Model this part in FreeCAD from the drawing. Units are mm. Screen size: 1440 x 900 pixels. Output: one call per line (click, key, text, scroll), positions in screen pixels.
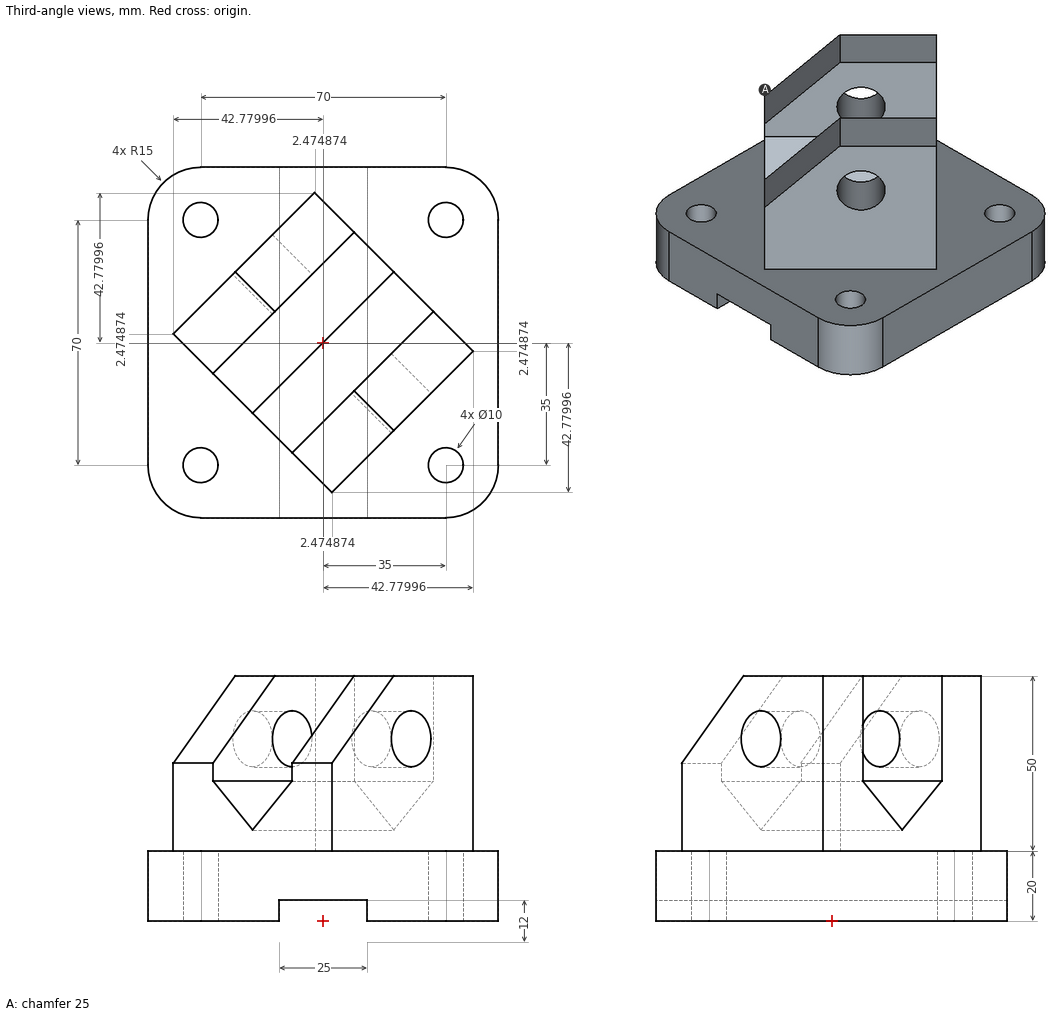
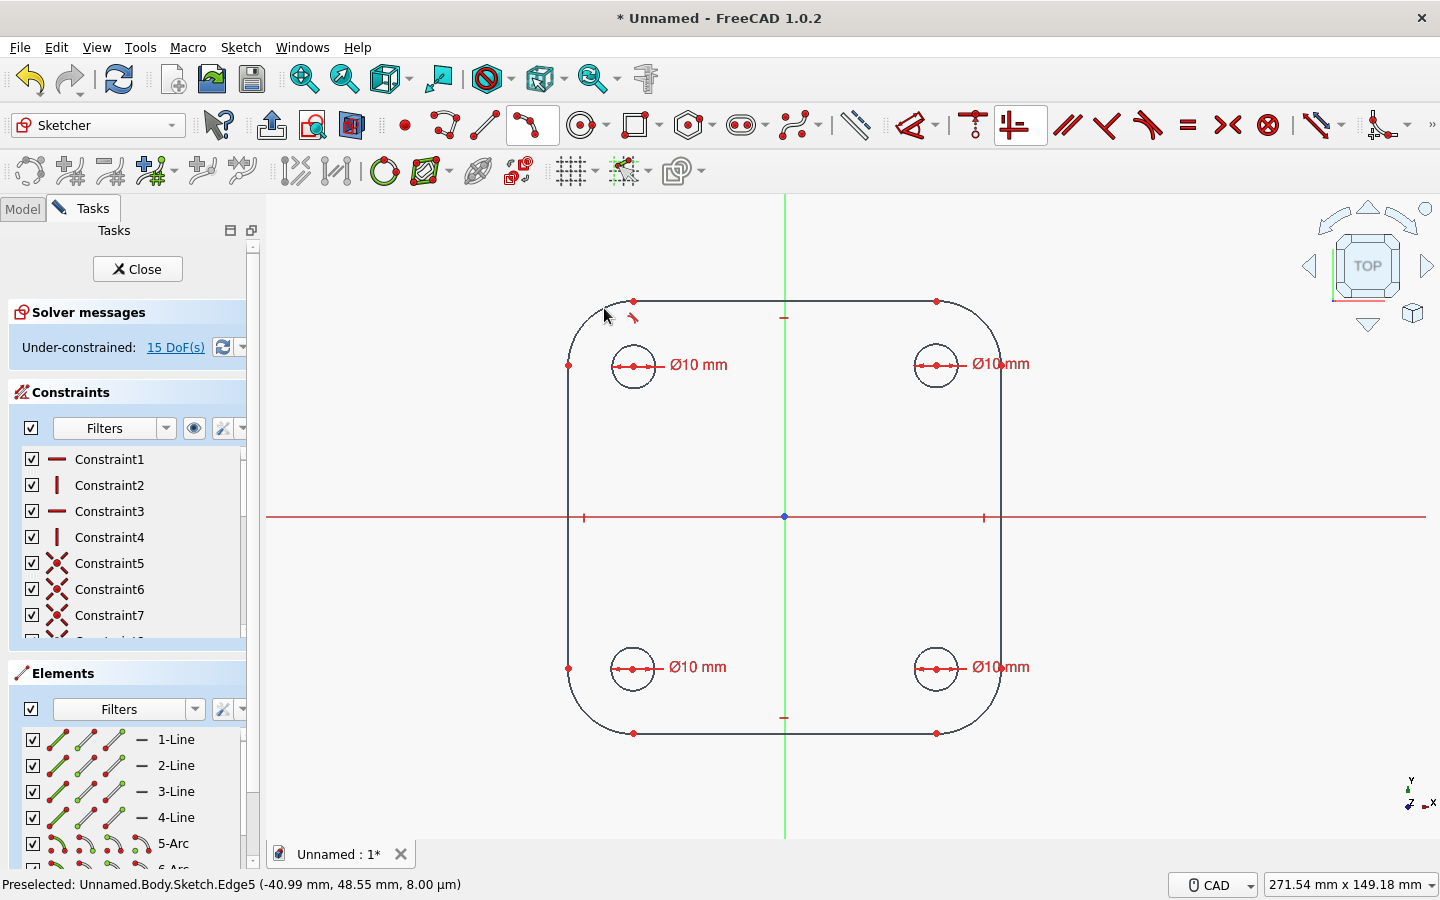
click(845, 301)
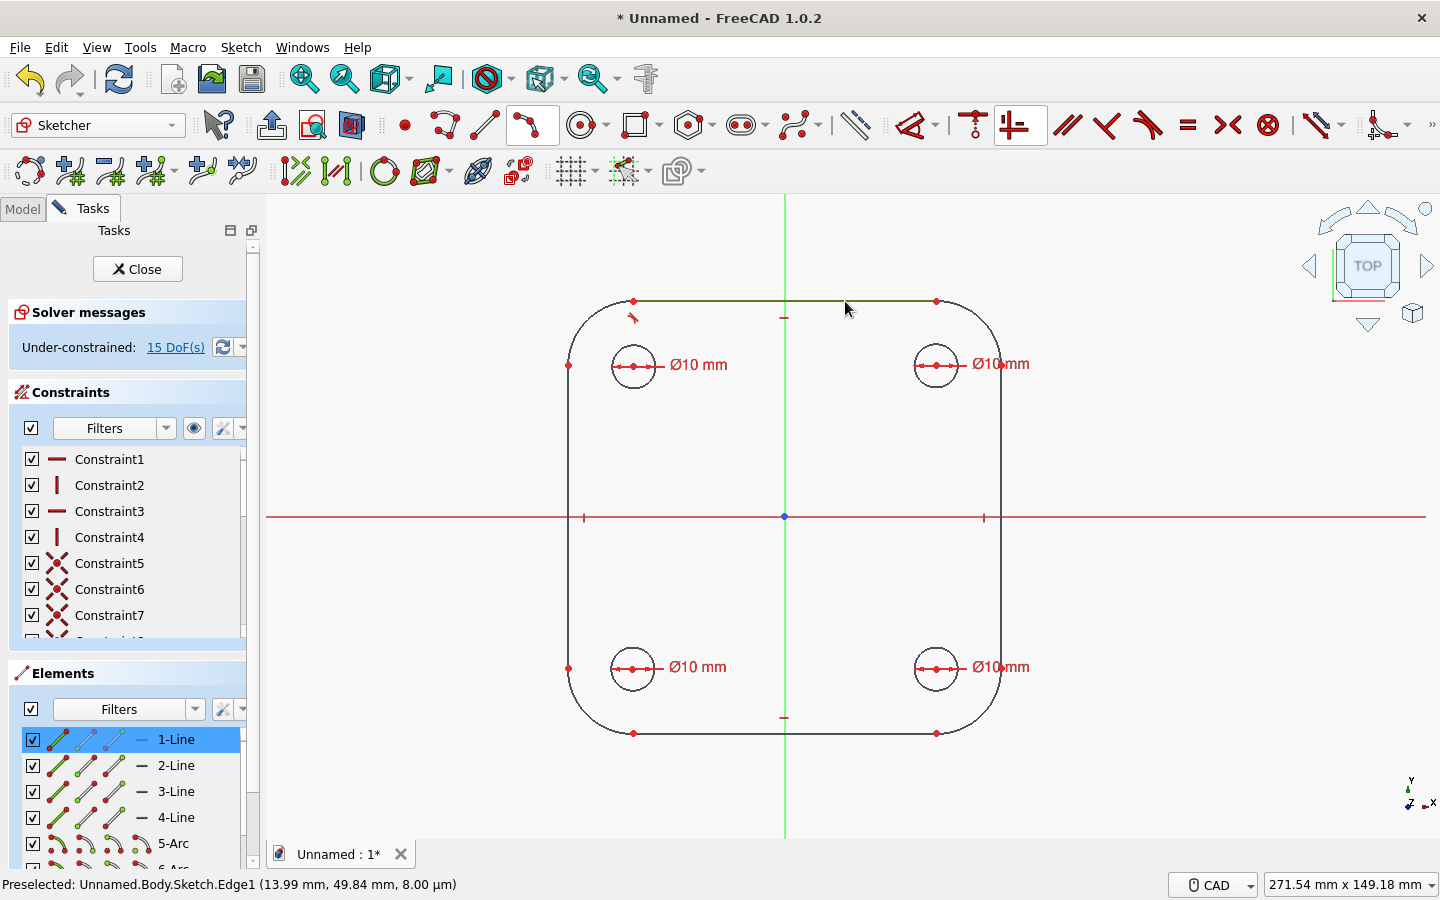
click(994, 336)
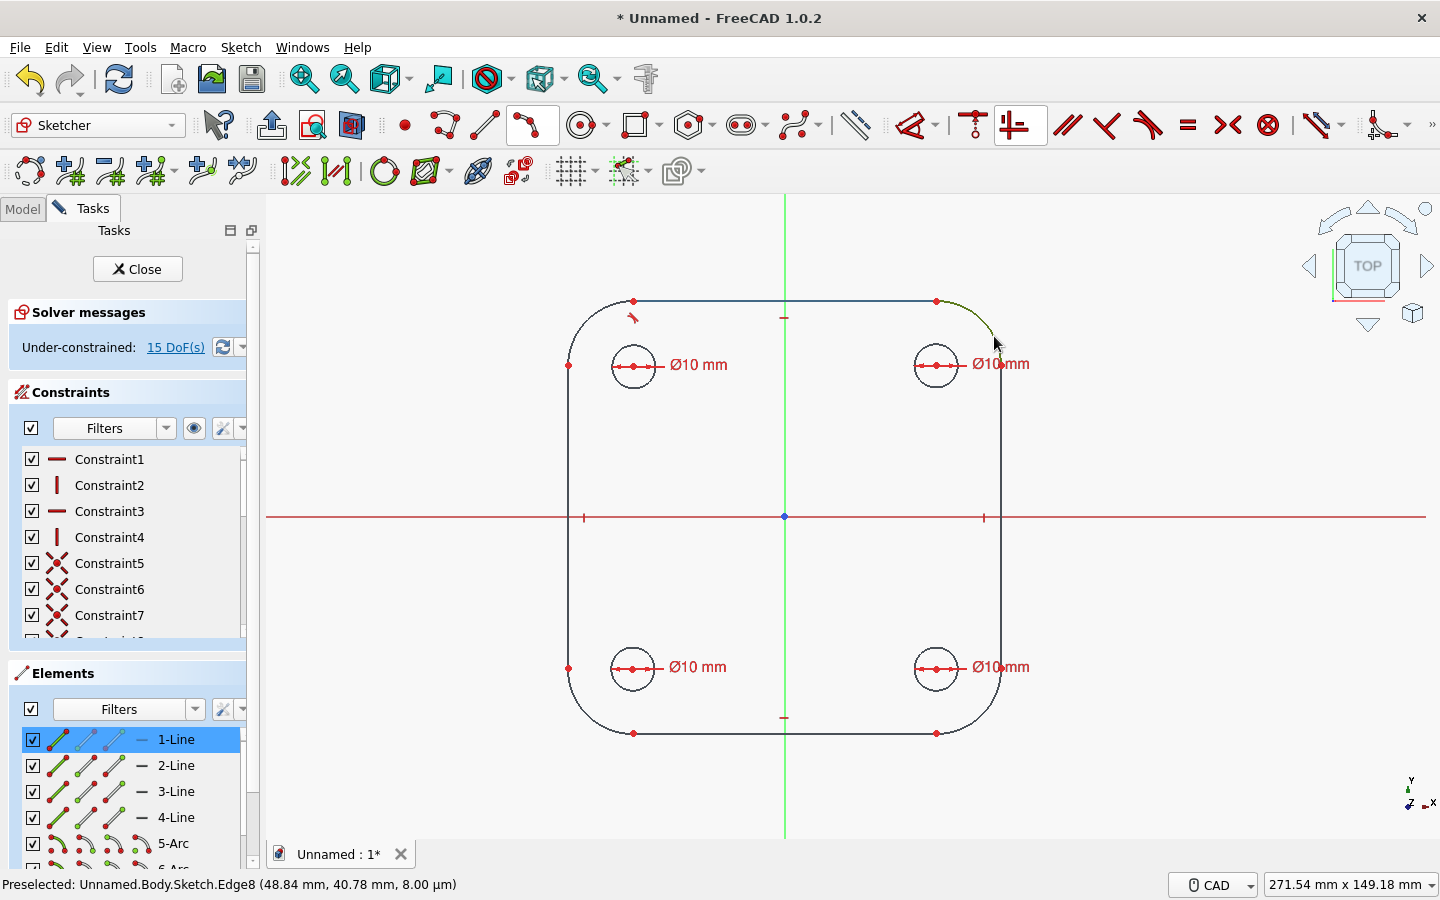
click(1148, 126)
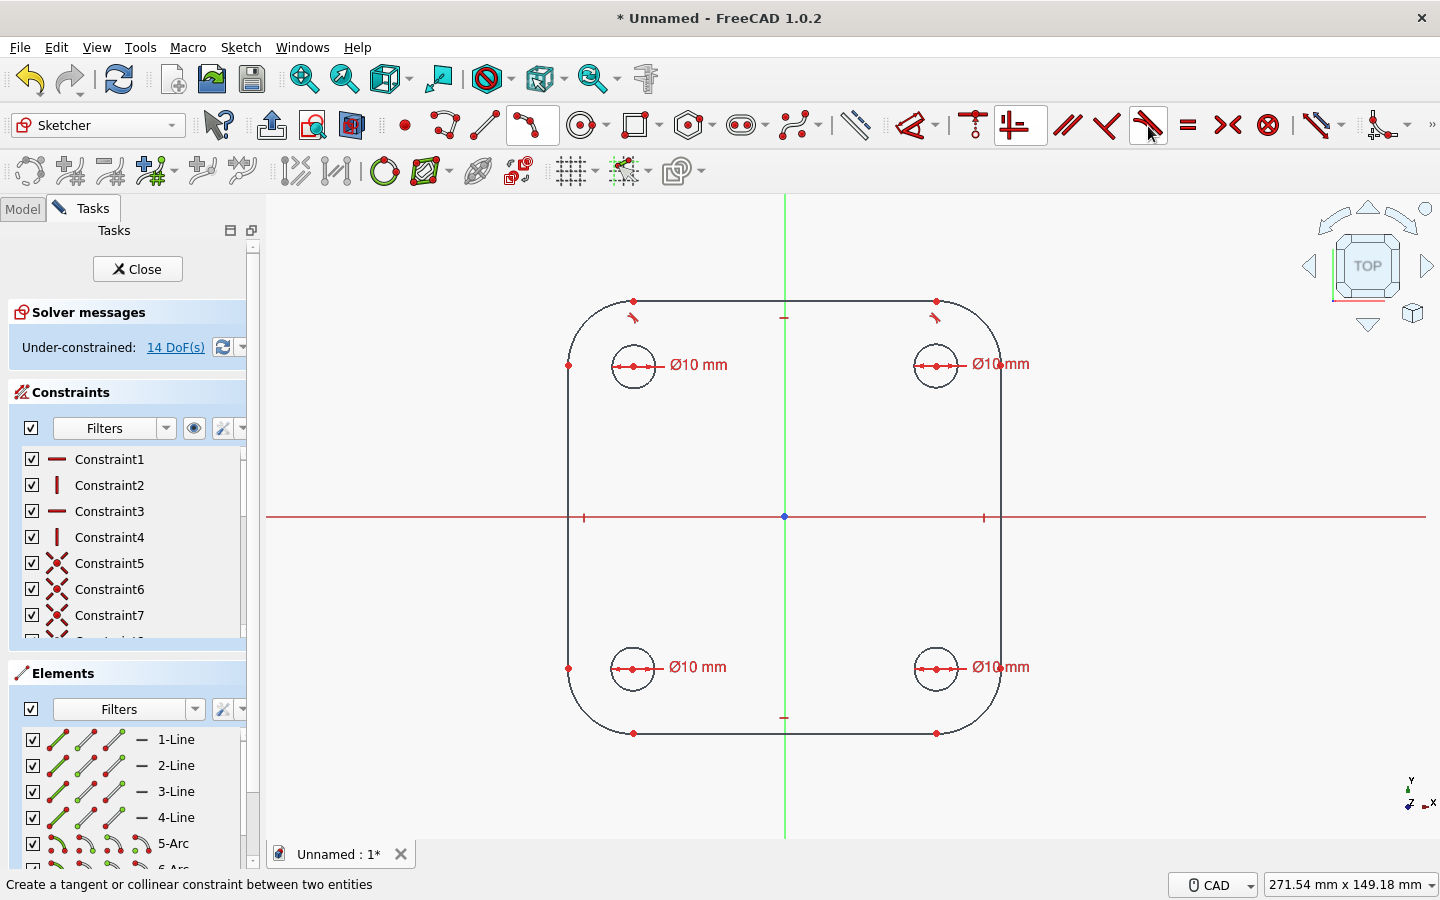
click(568, 457)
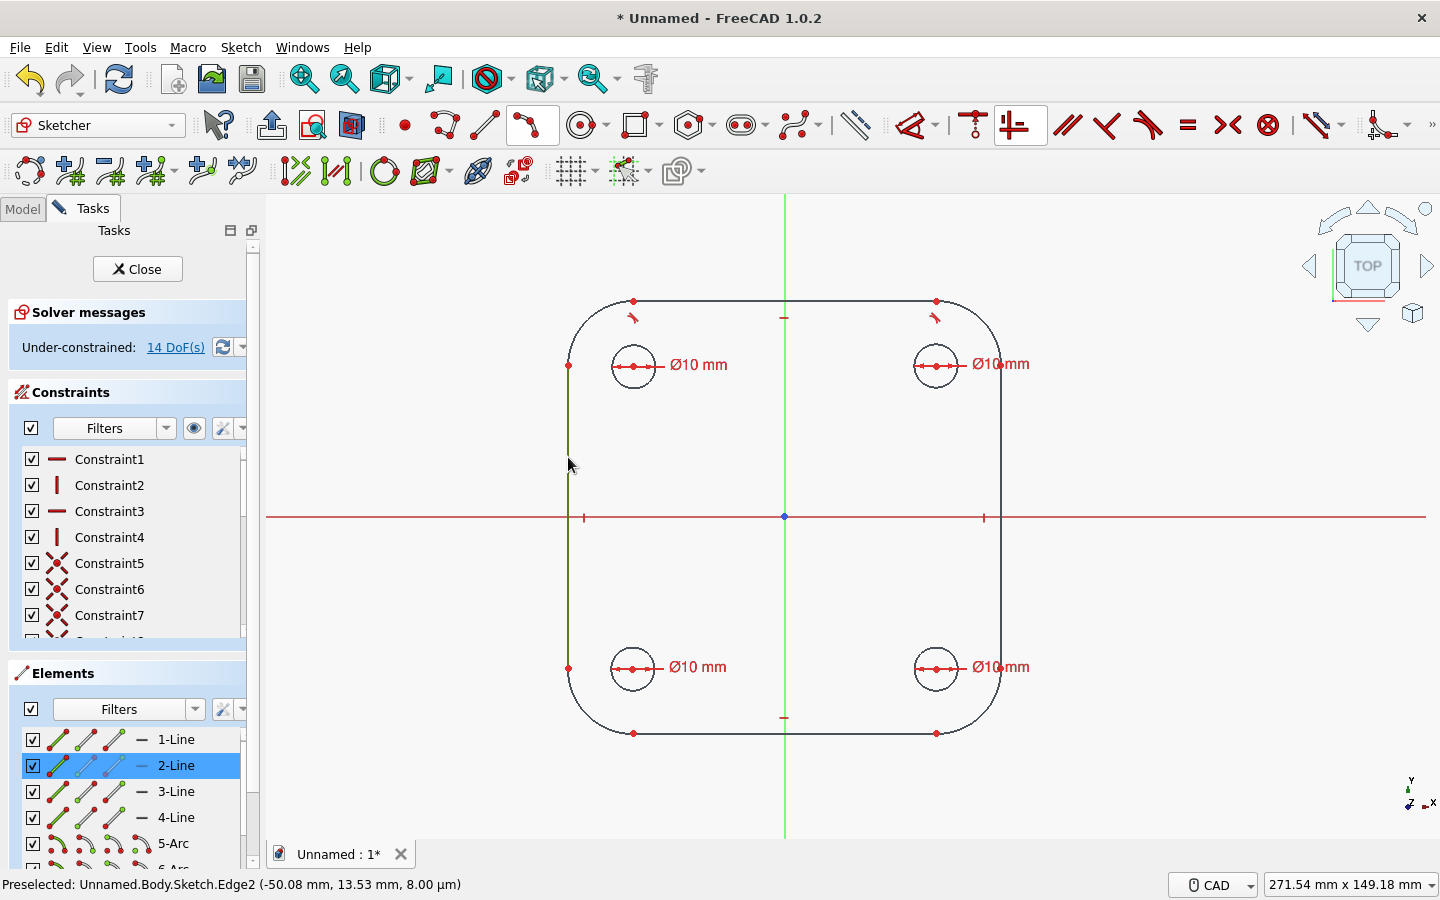
click(604, 308)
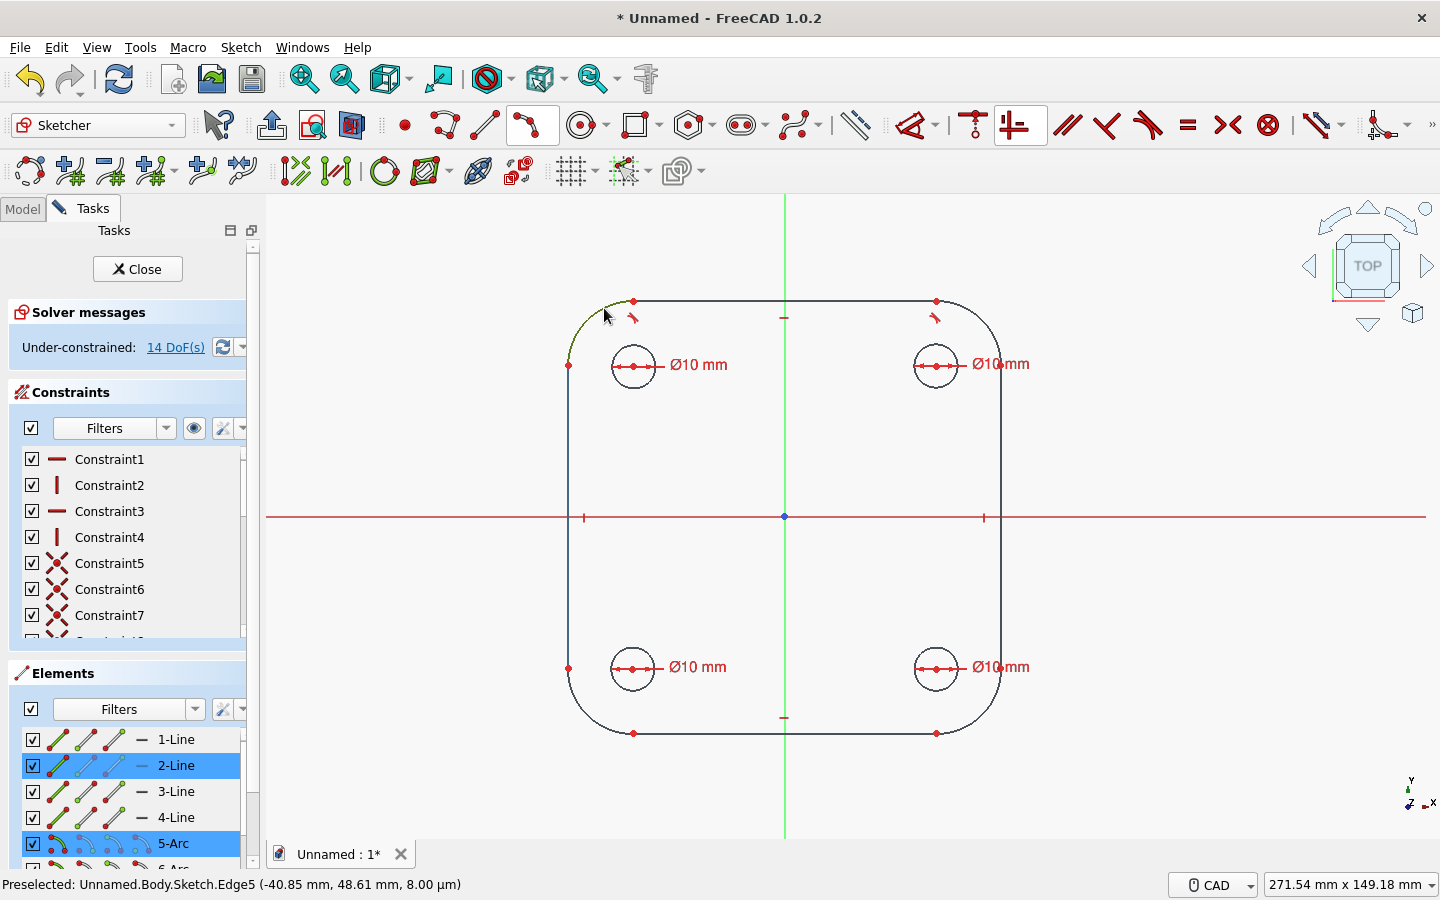
click(1148, 126)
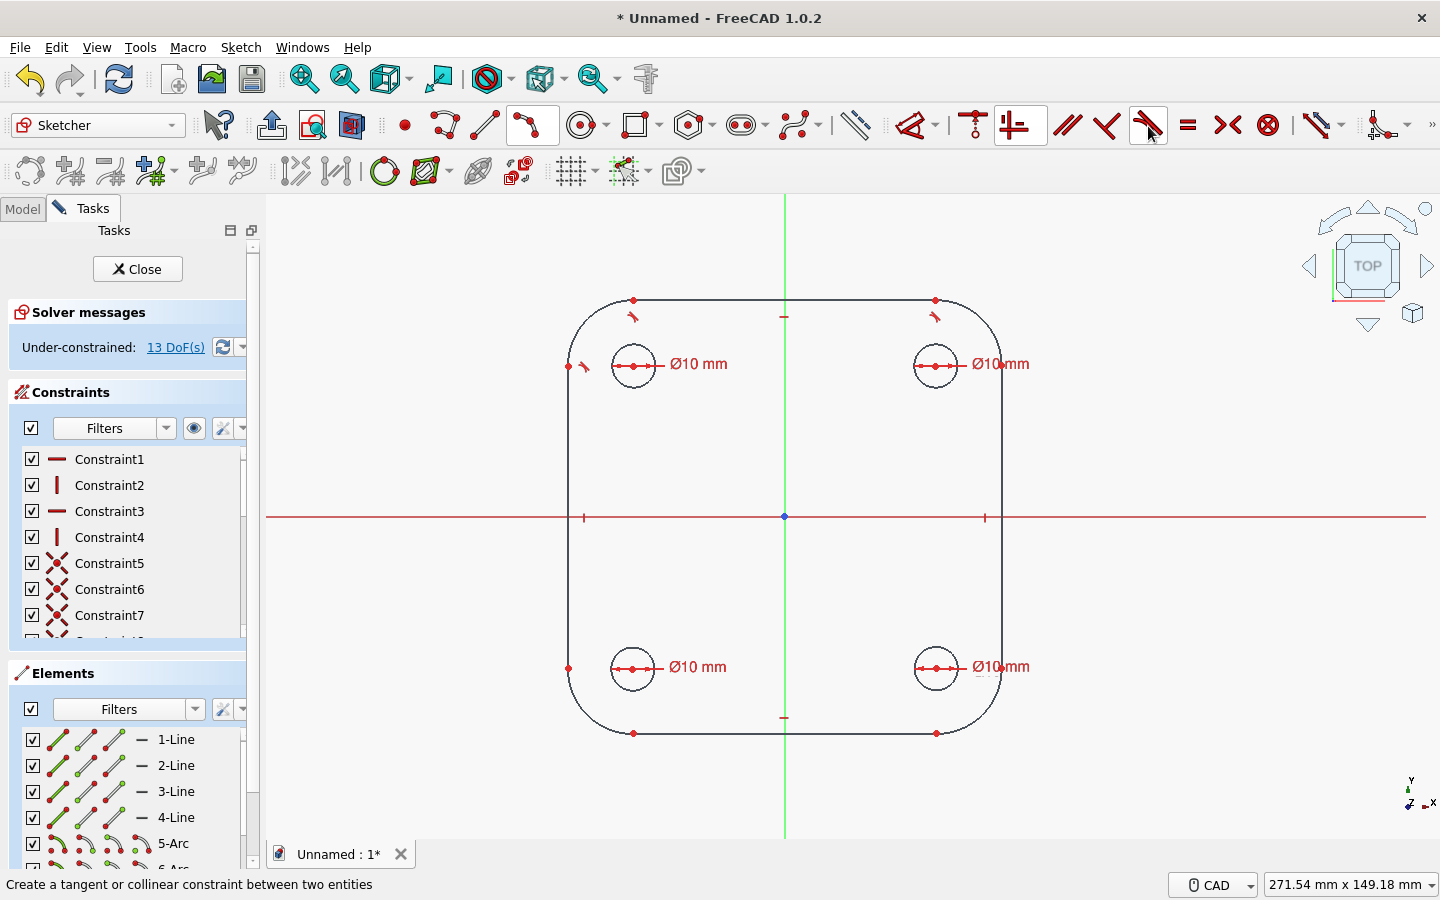
click(568, 457)